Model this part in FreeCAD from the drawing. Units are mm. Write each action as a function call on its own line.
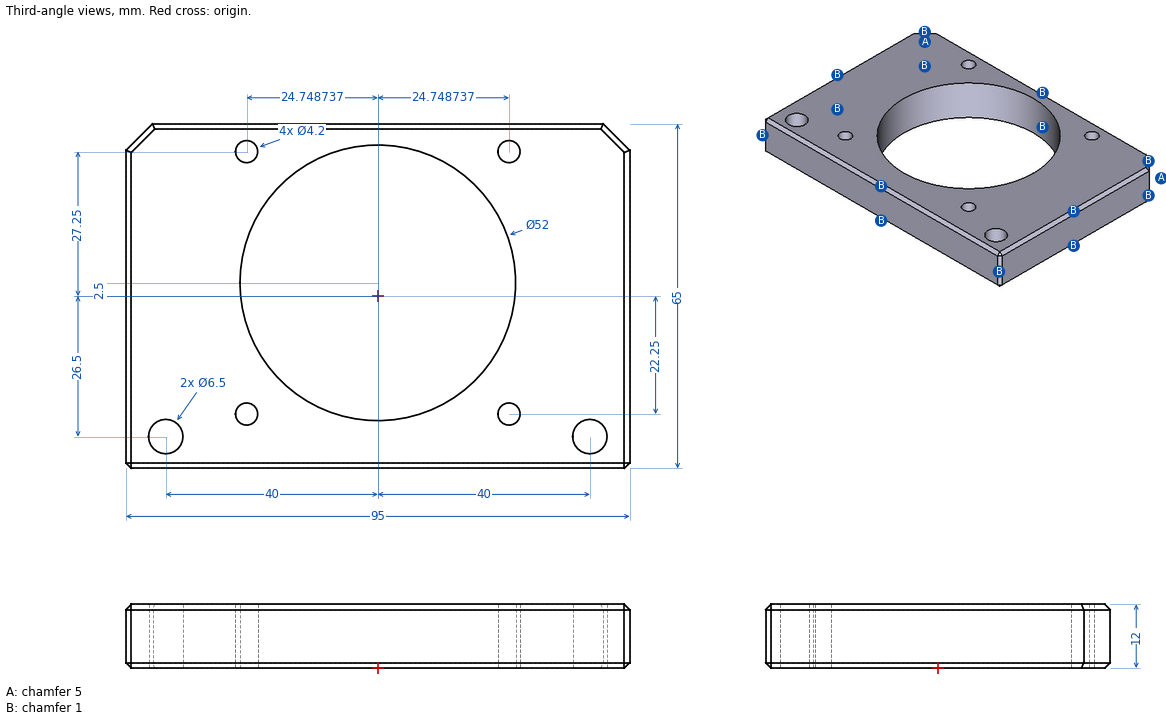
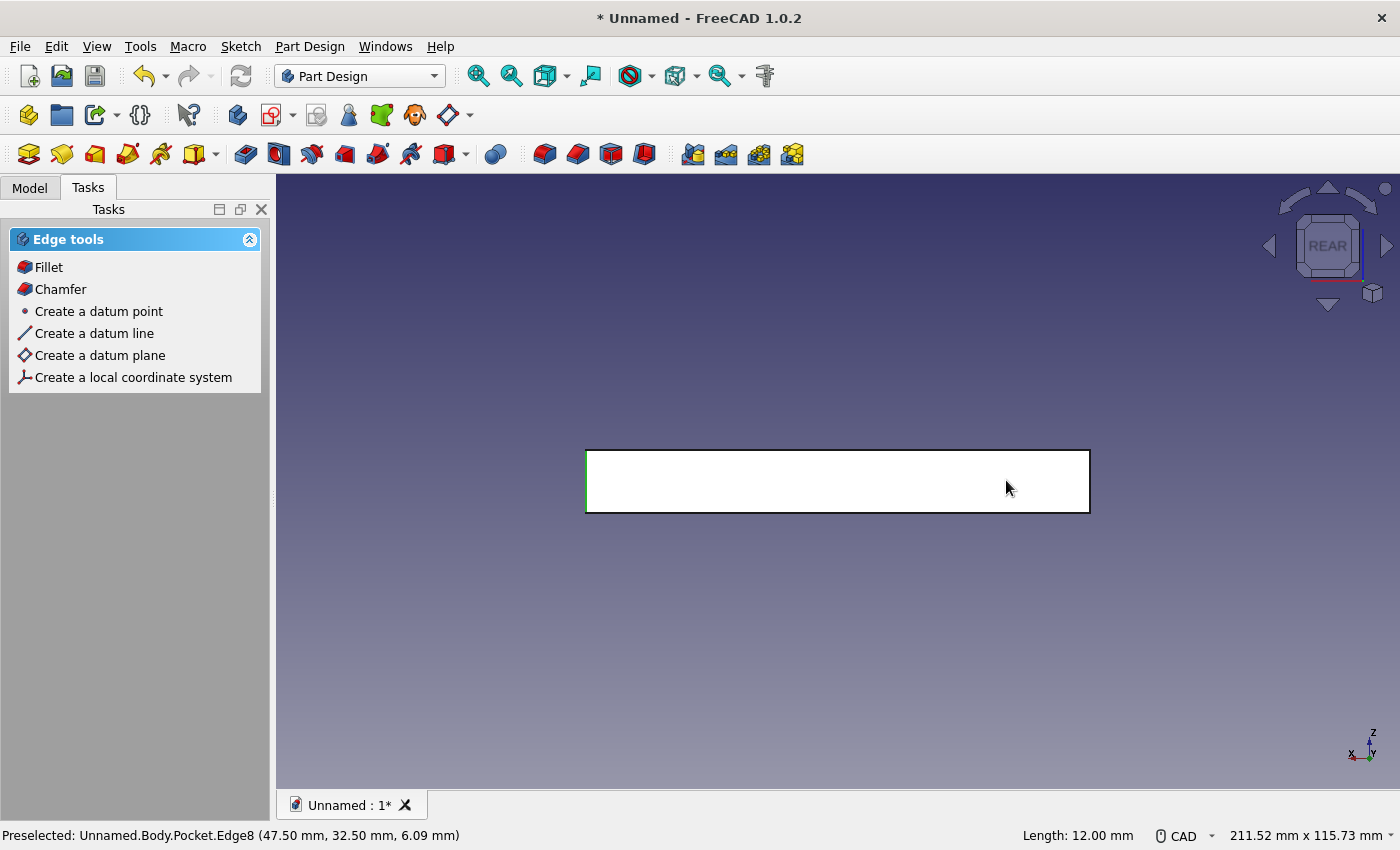
click(479, 76)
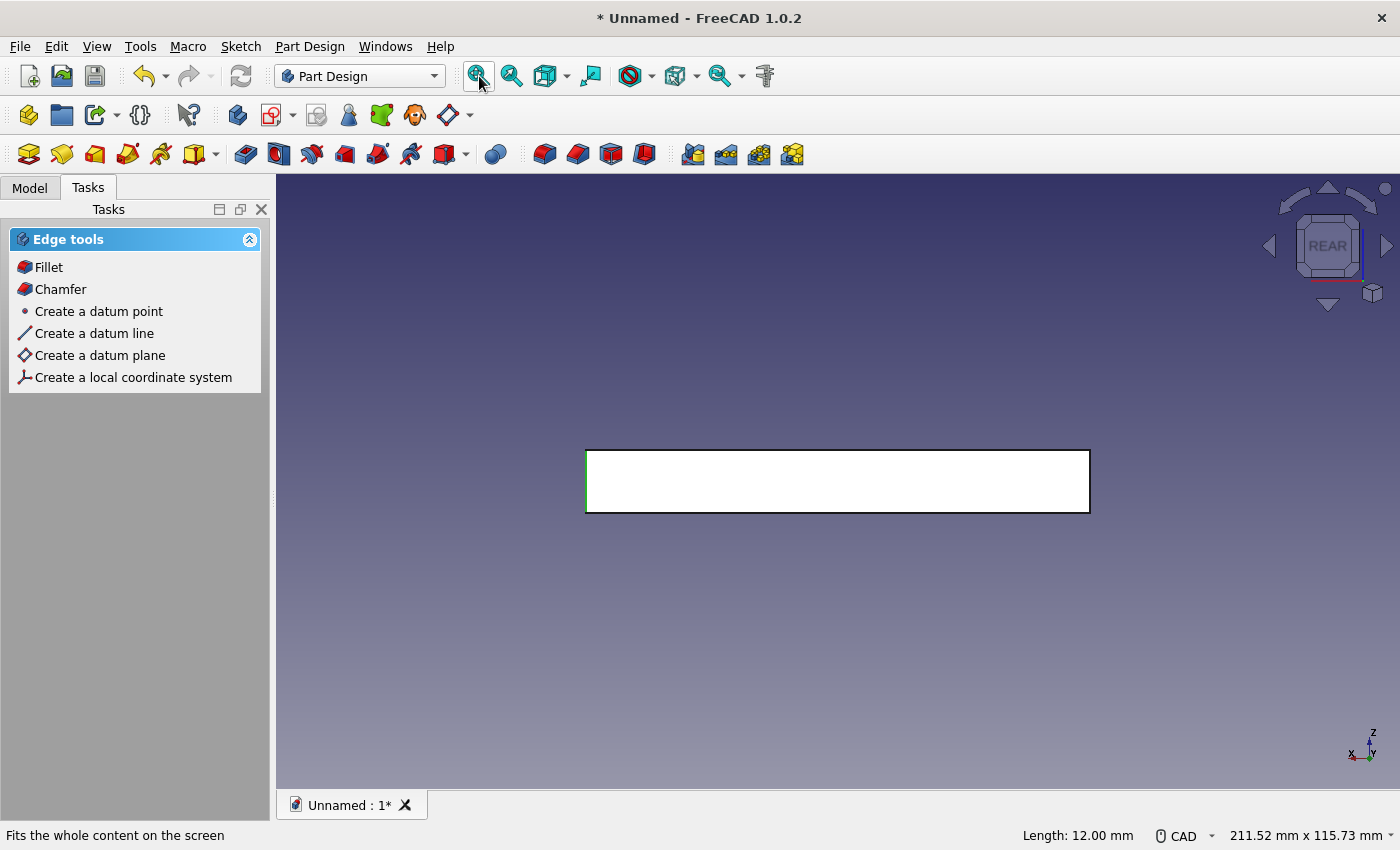
click(1090, 481, ctrl)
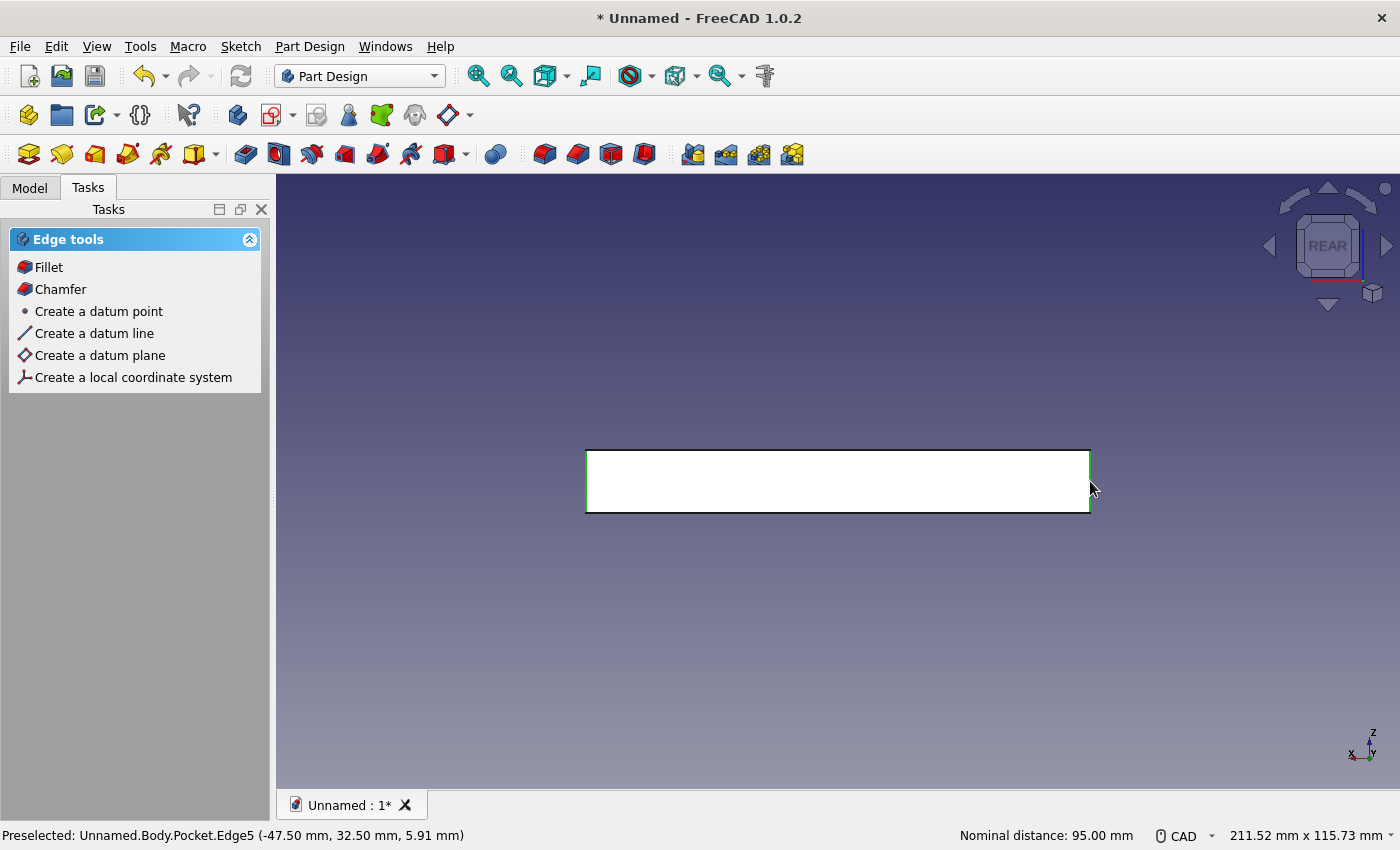
click(578, 154)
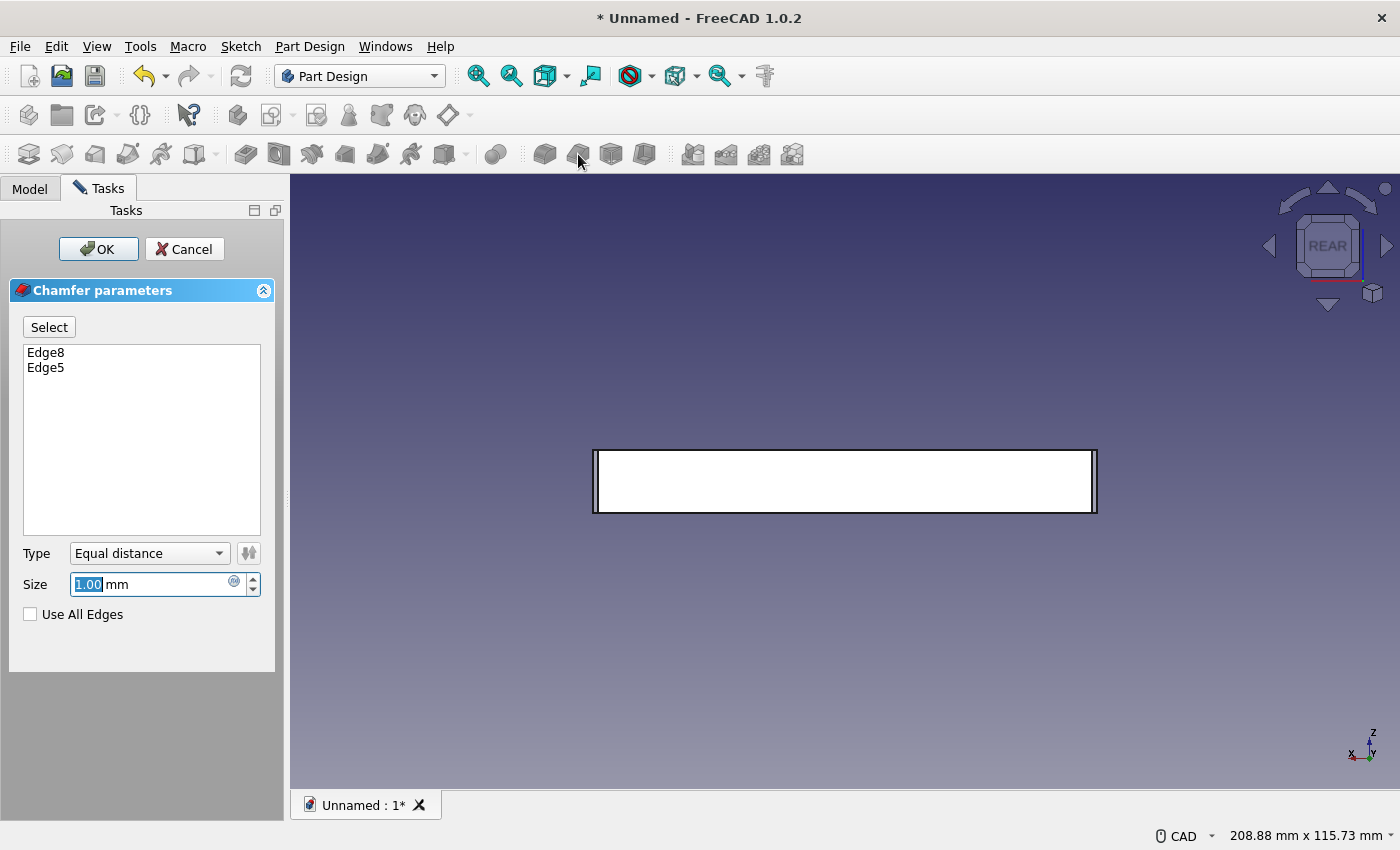
text(5)
key(Tab)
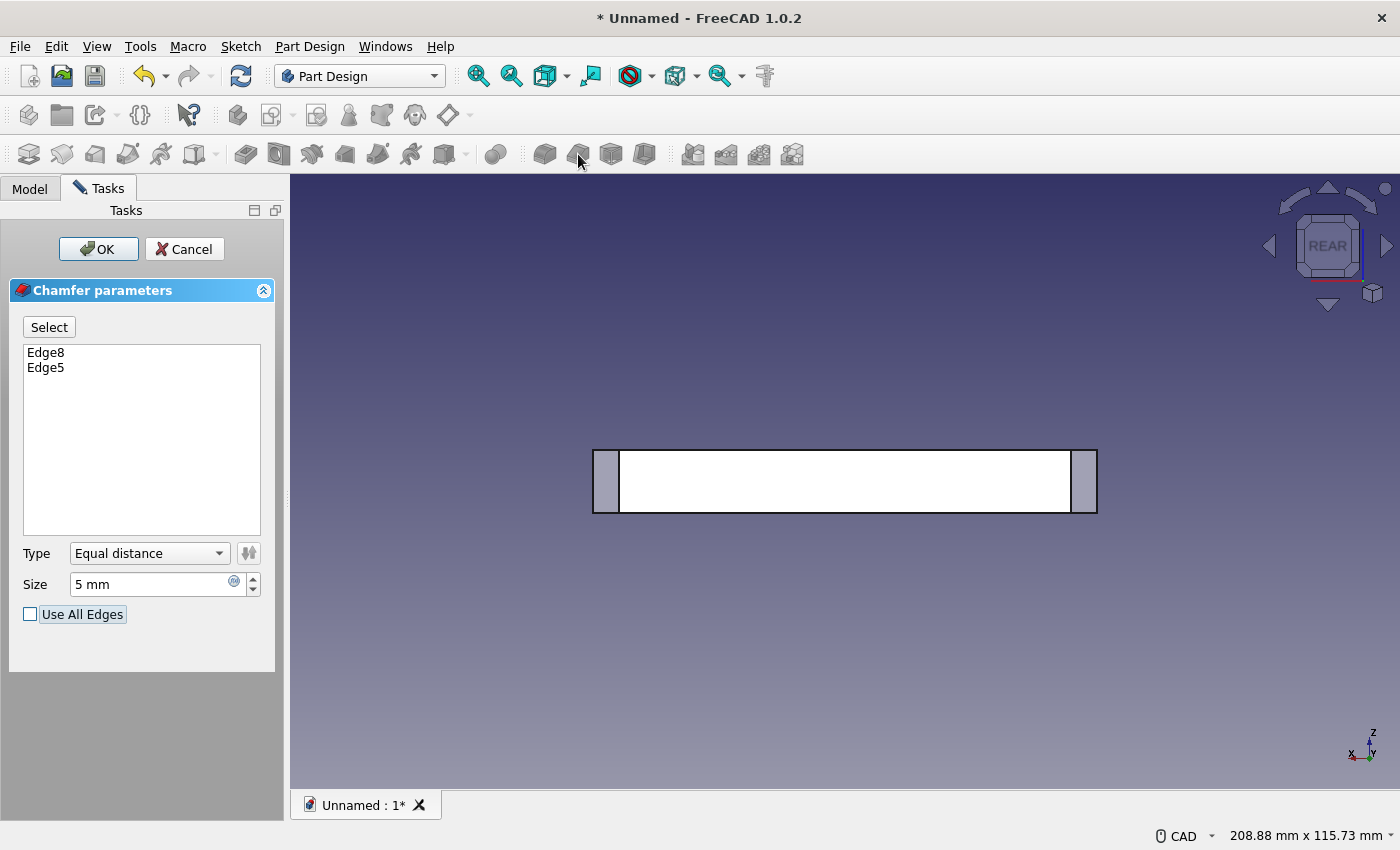
click(99, 249)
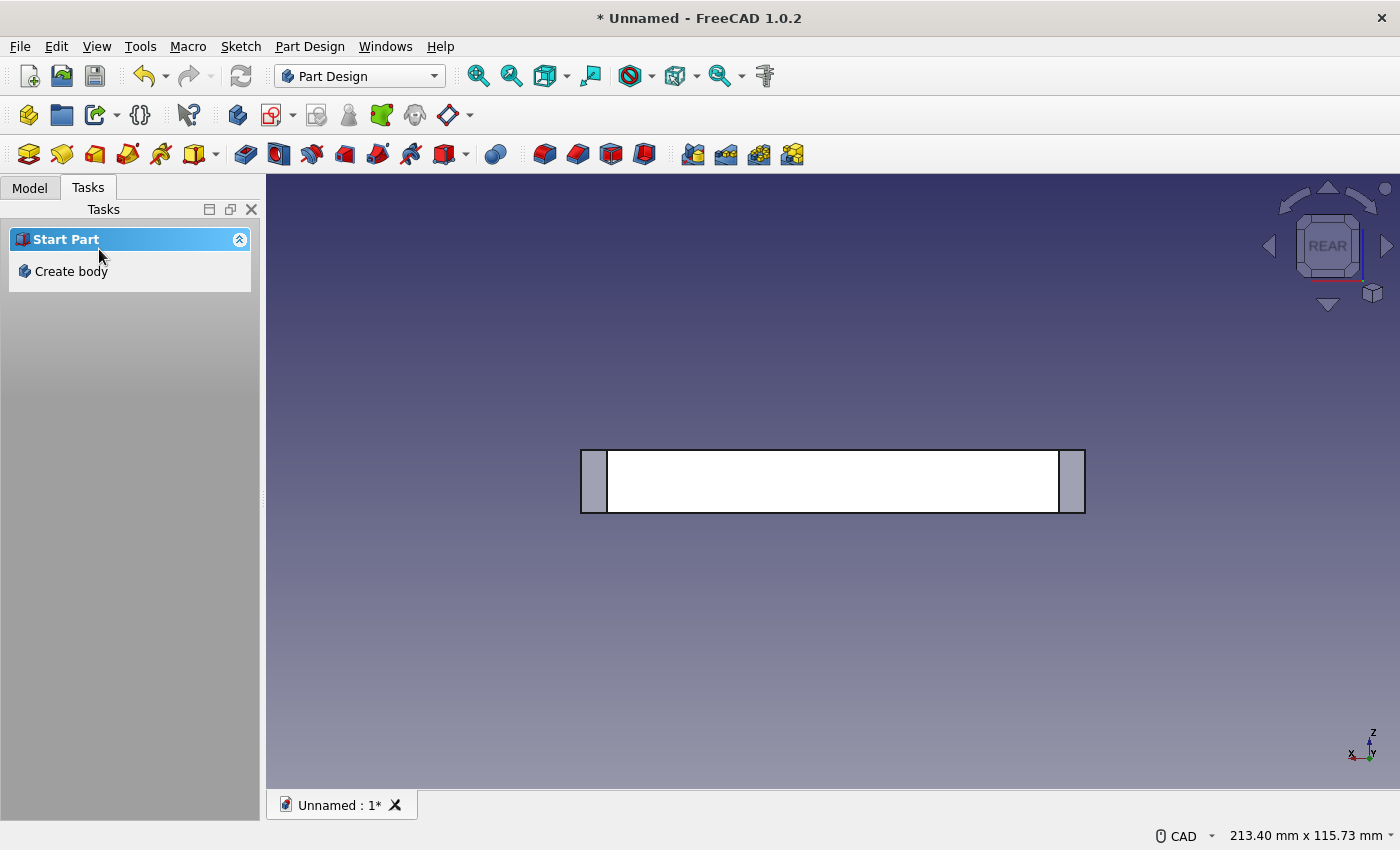
click(479, 76)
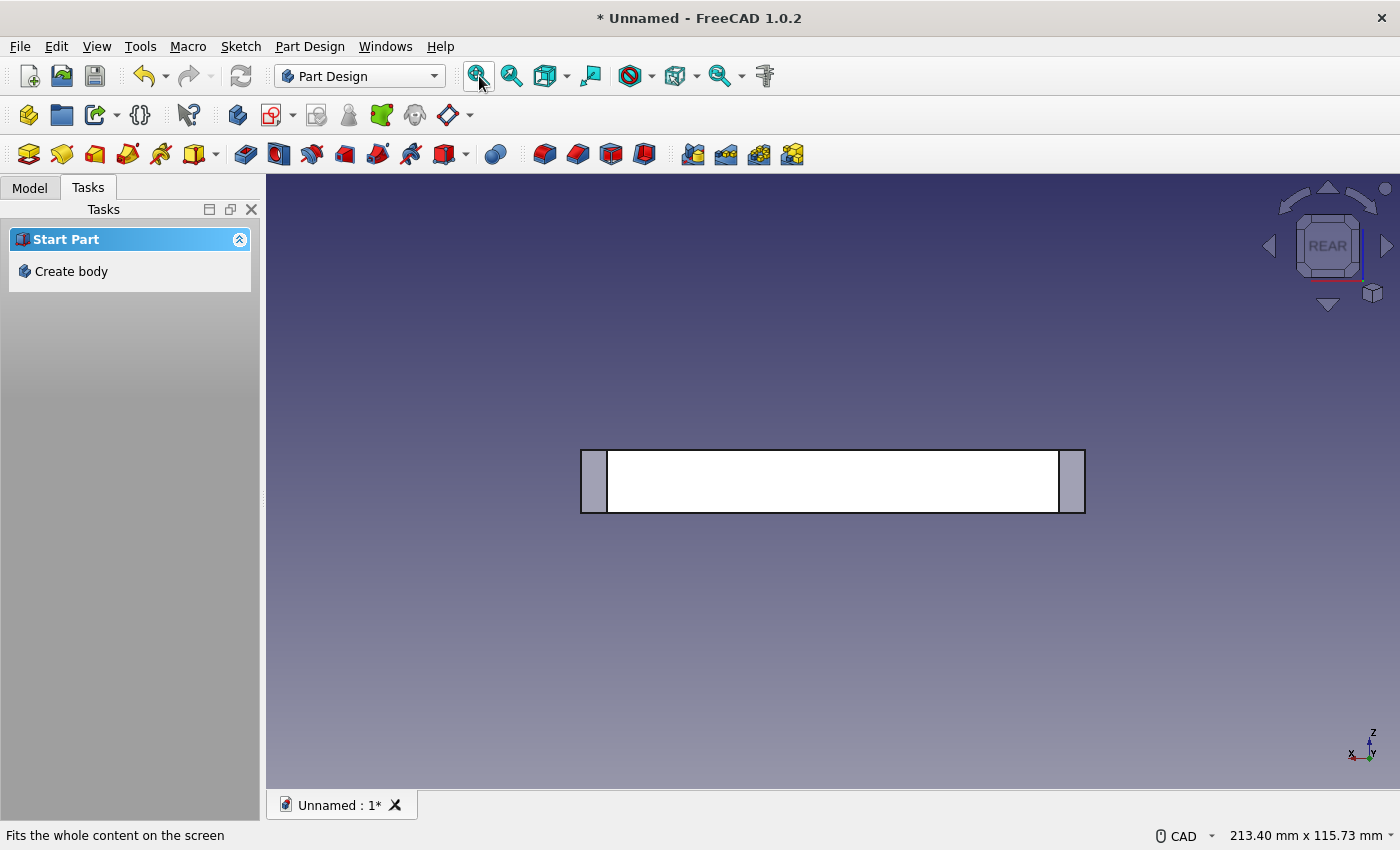
click(270, 116)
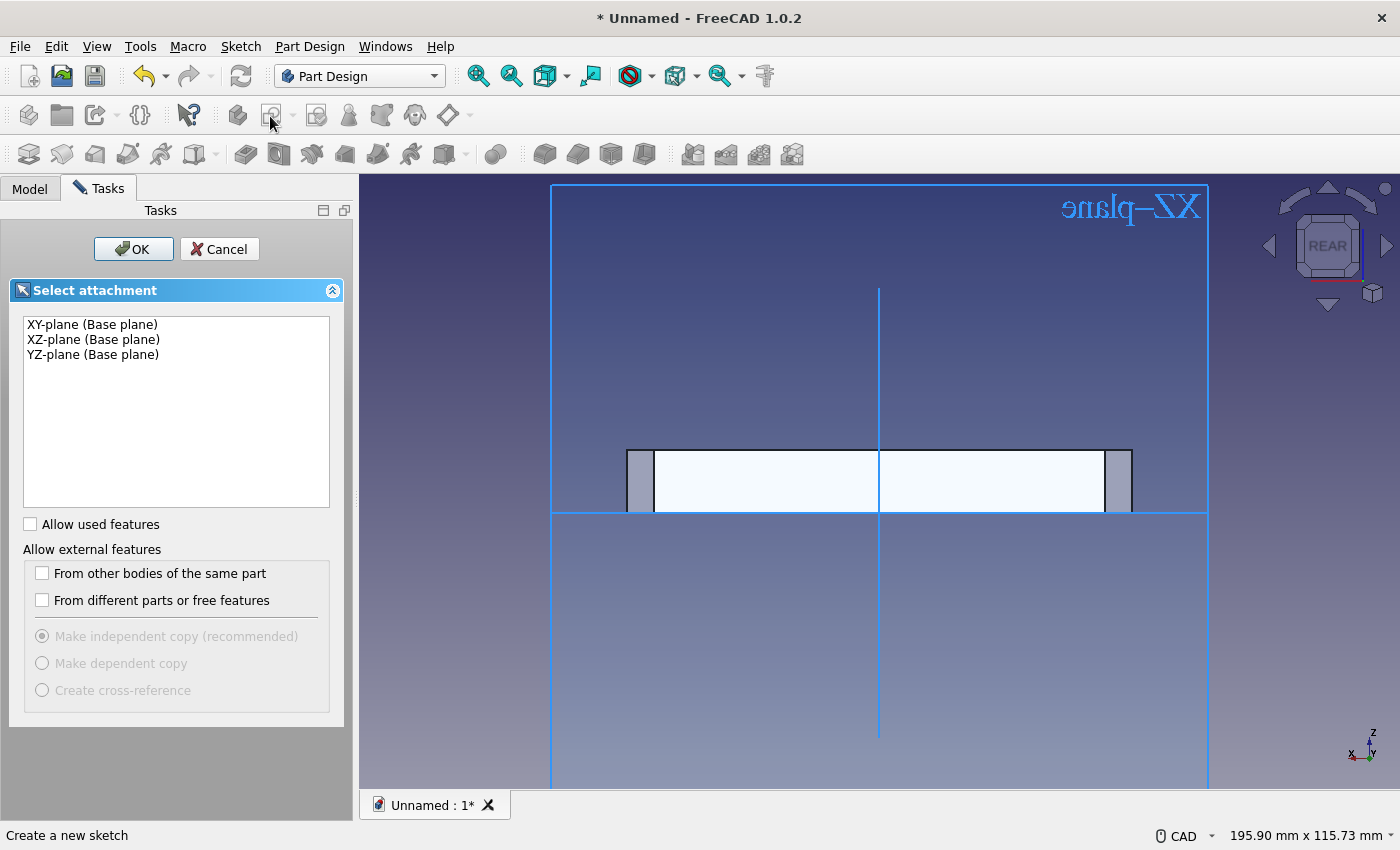
click(84, 324)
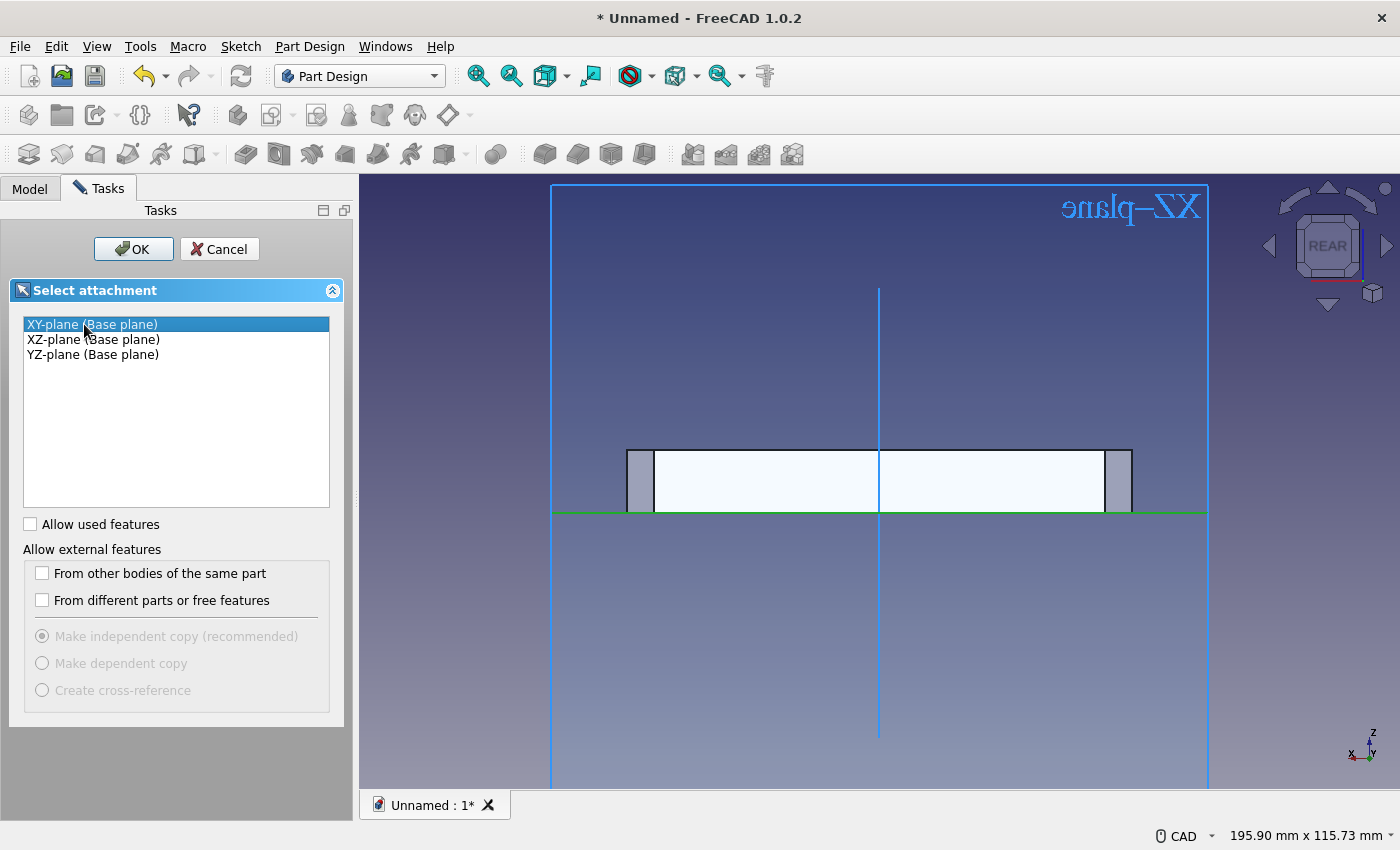
click(134, 249)